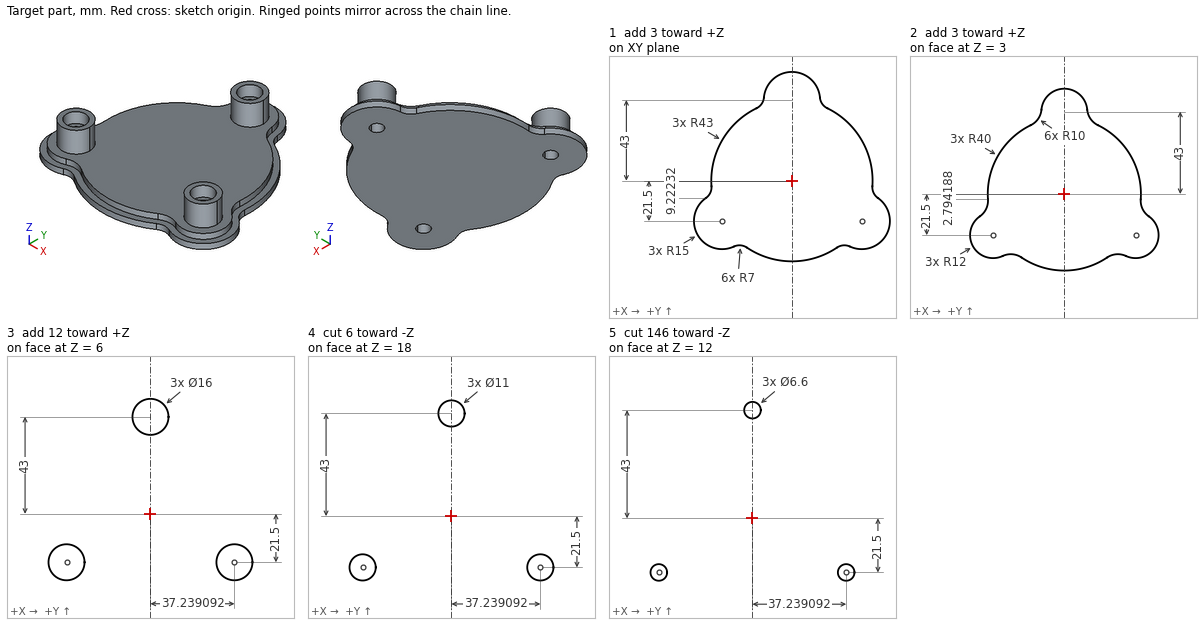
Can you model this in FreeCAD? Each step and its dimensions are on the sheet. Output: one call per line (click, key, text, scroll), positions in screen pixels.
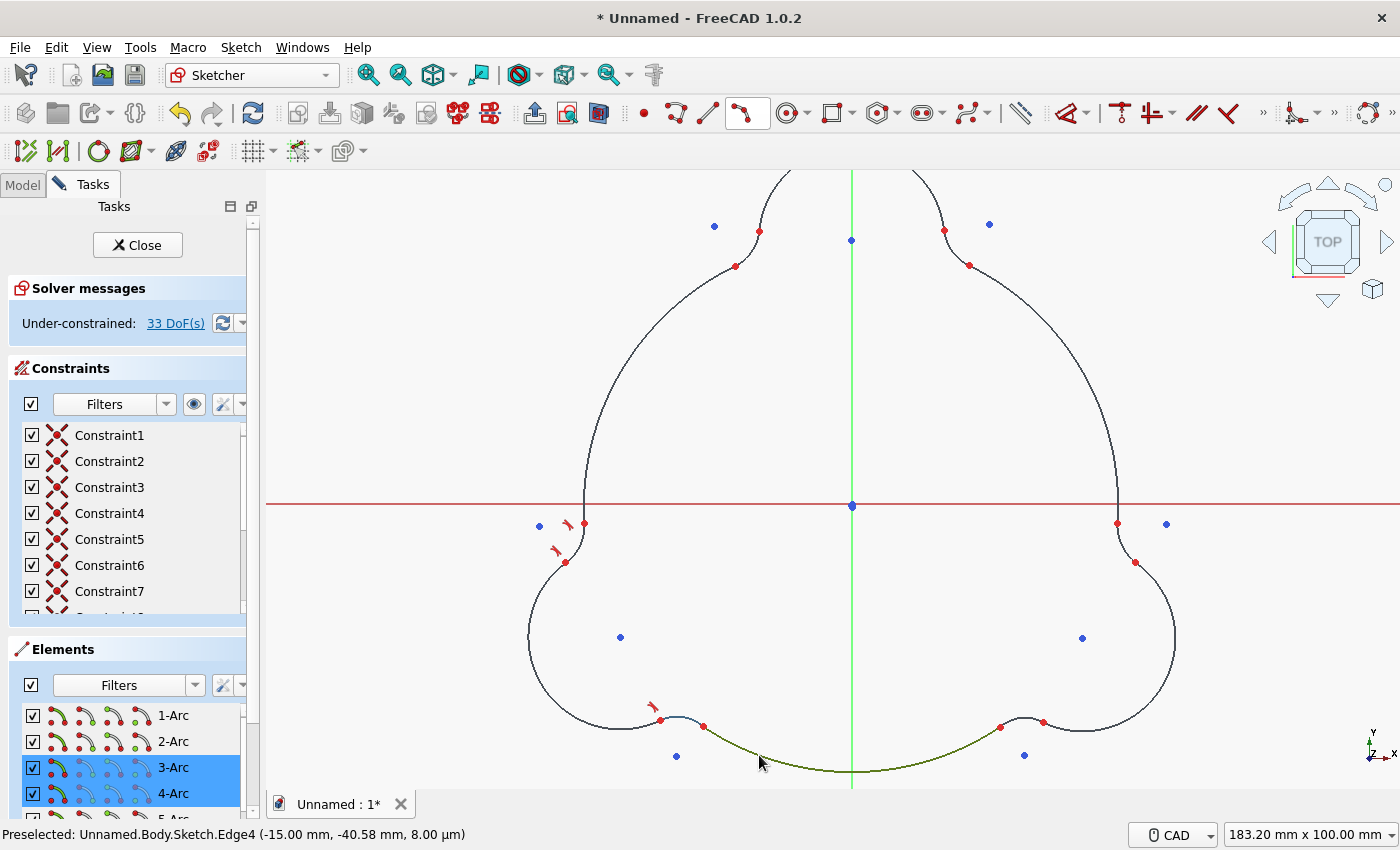
key(t)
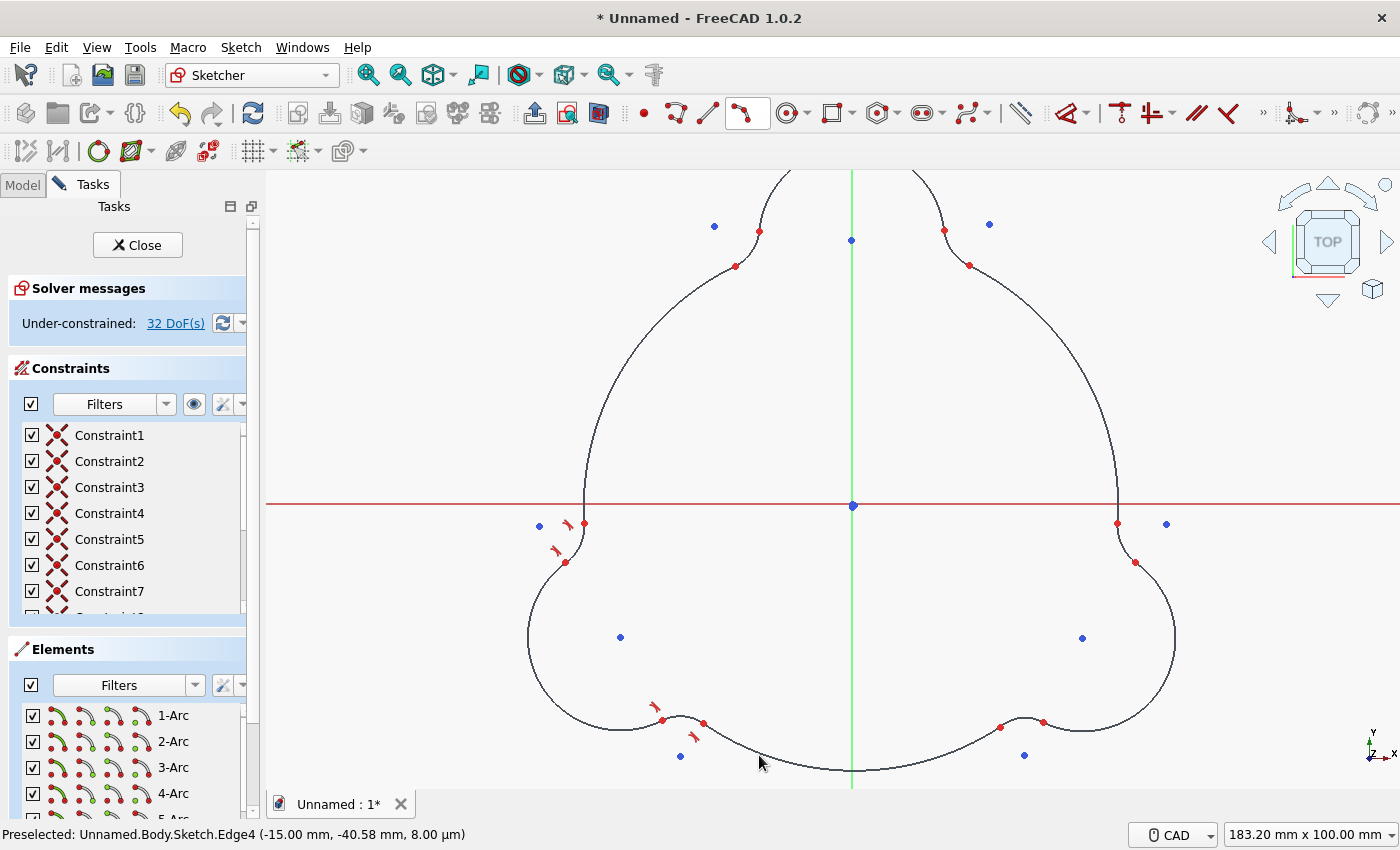
click(759, 753)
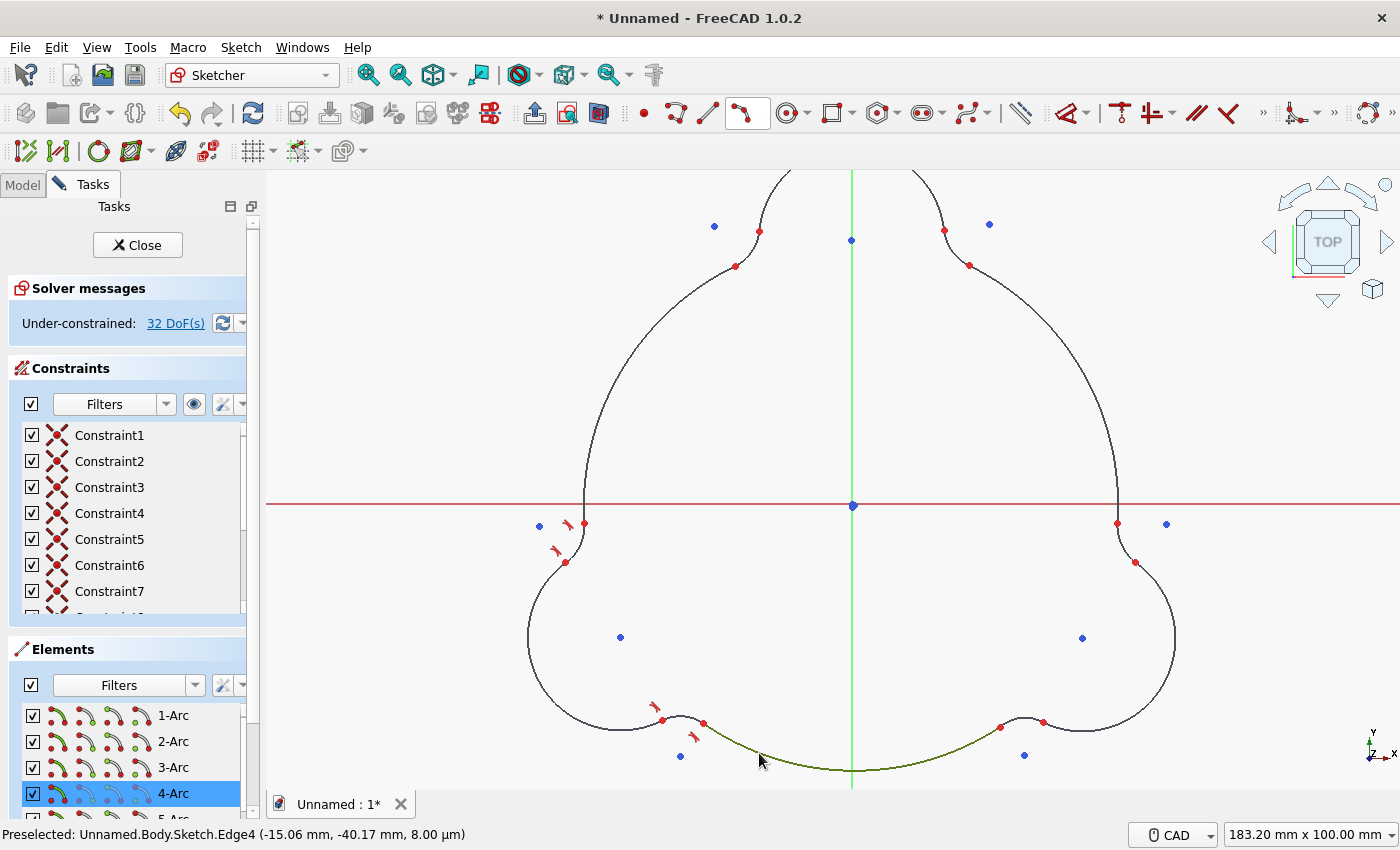
click(1030, 718)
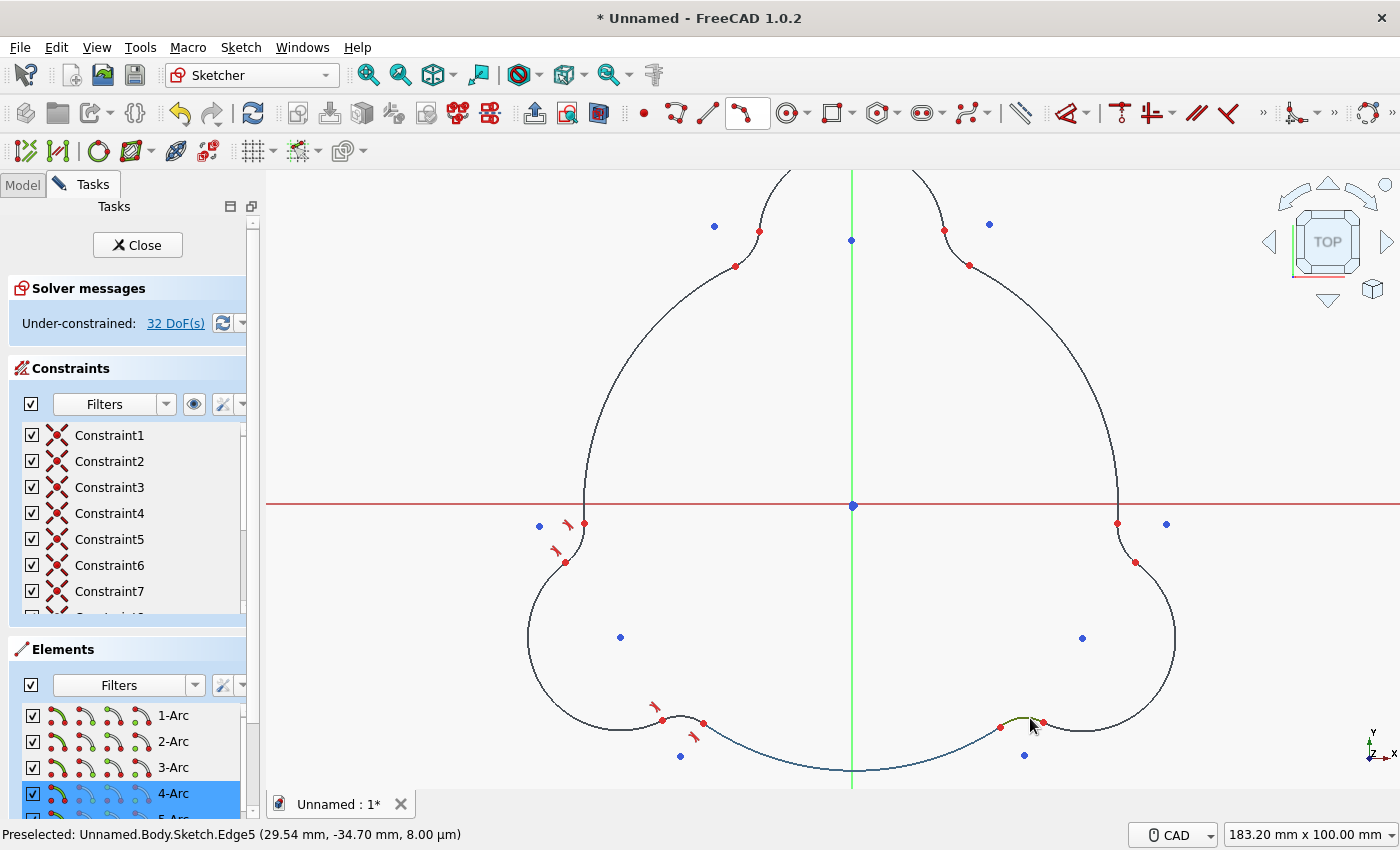
key(t)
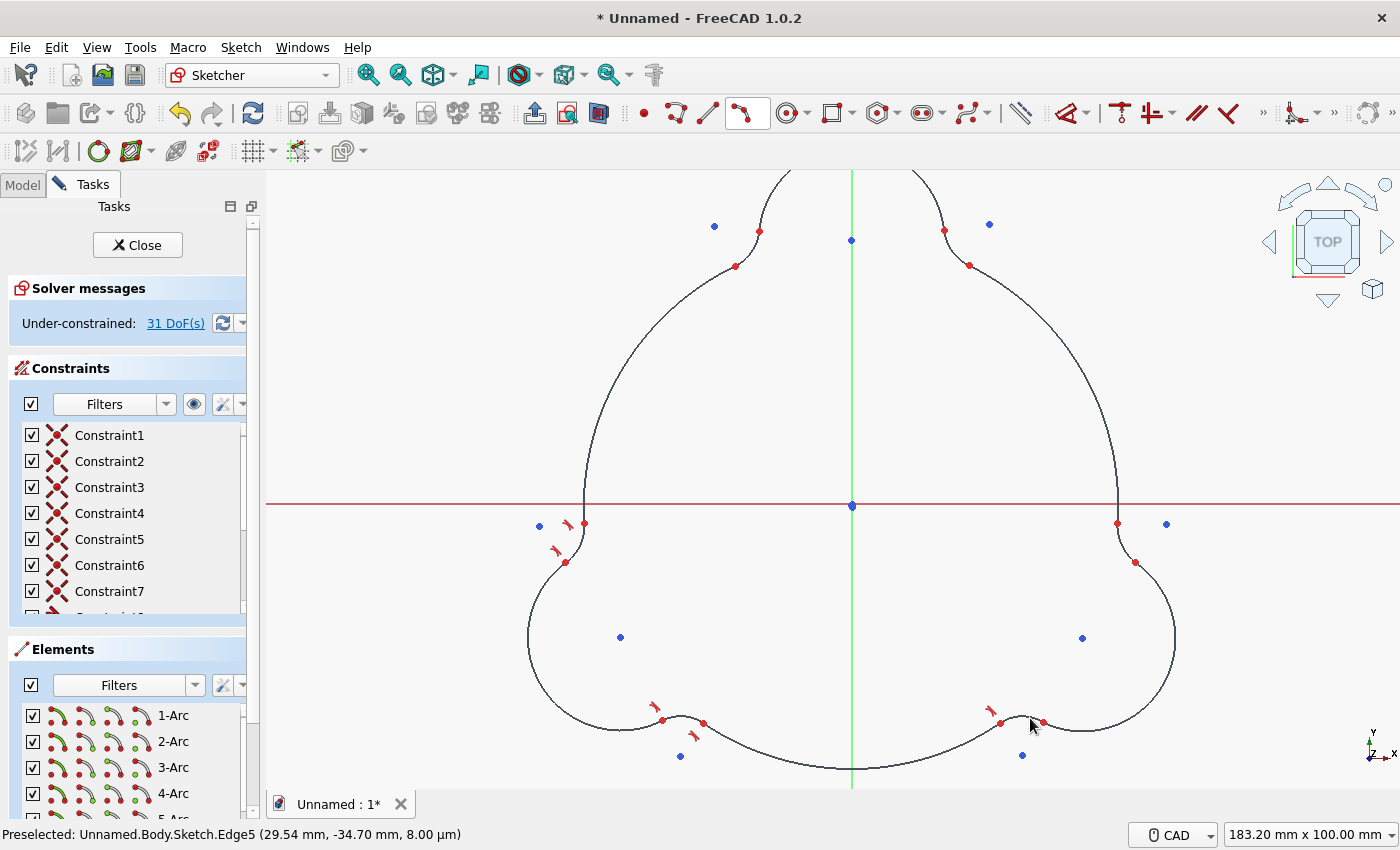
click(1031, 717)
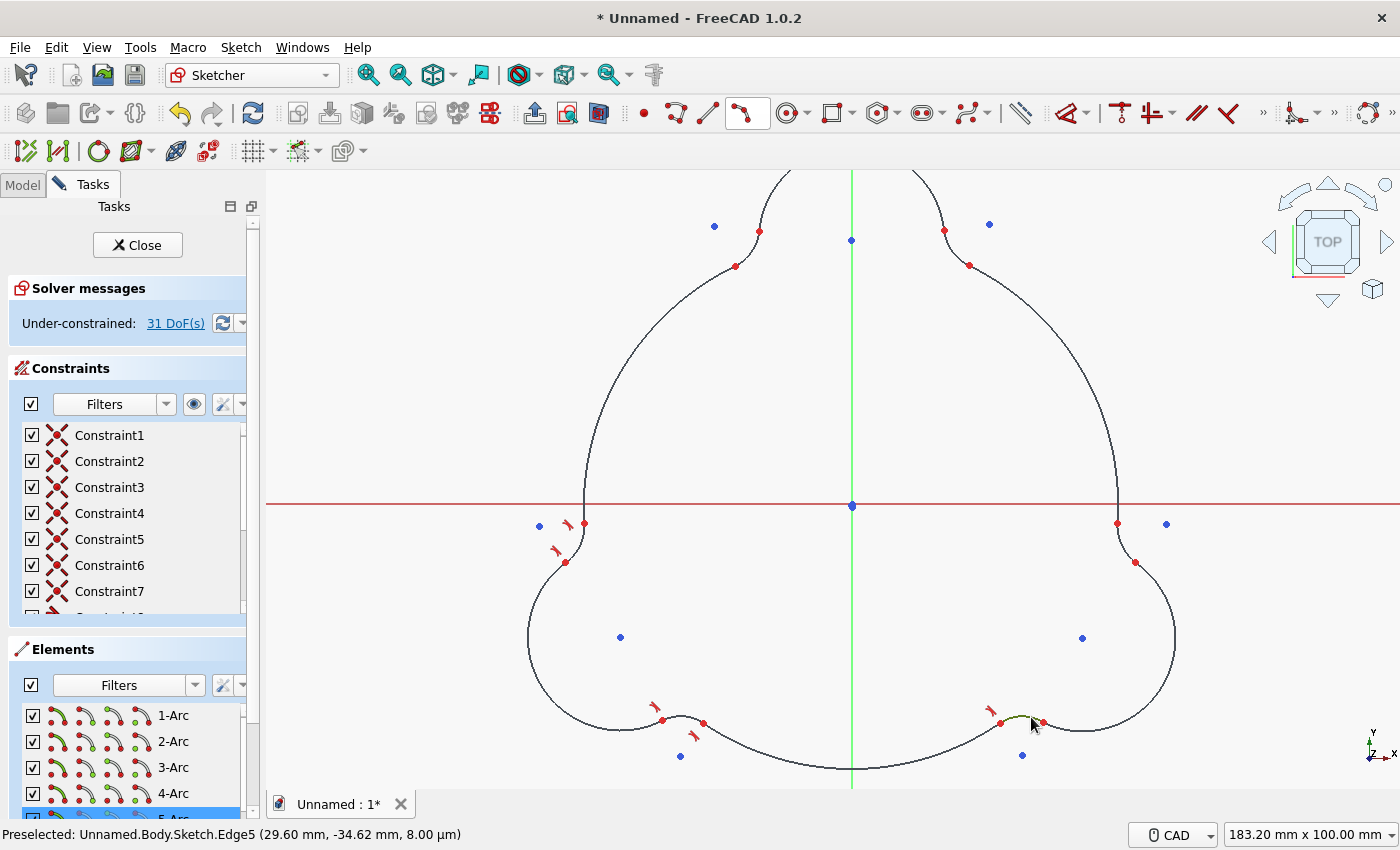
click(1123, 722)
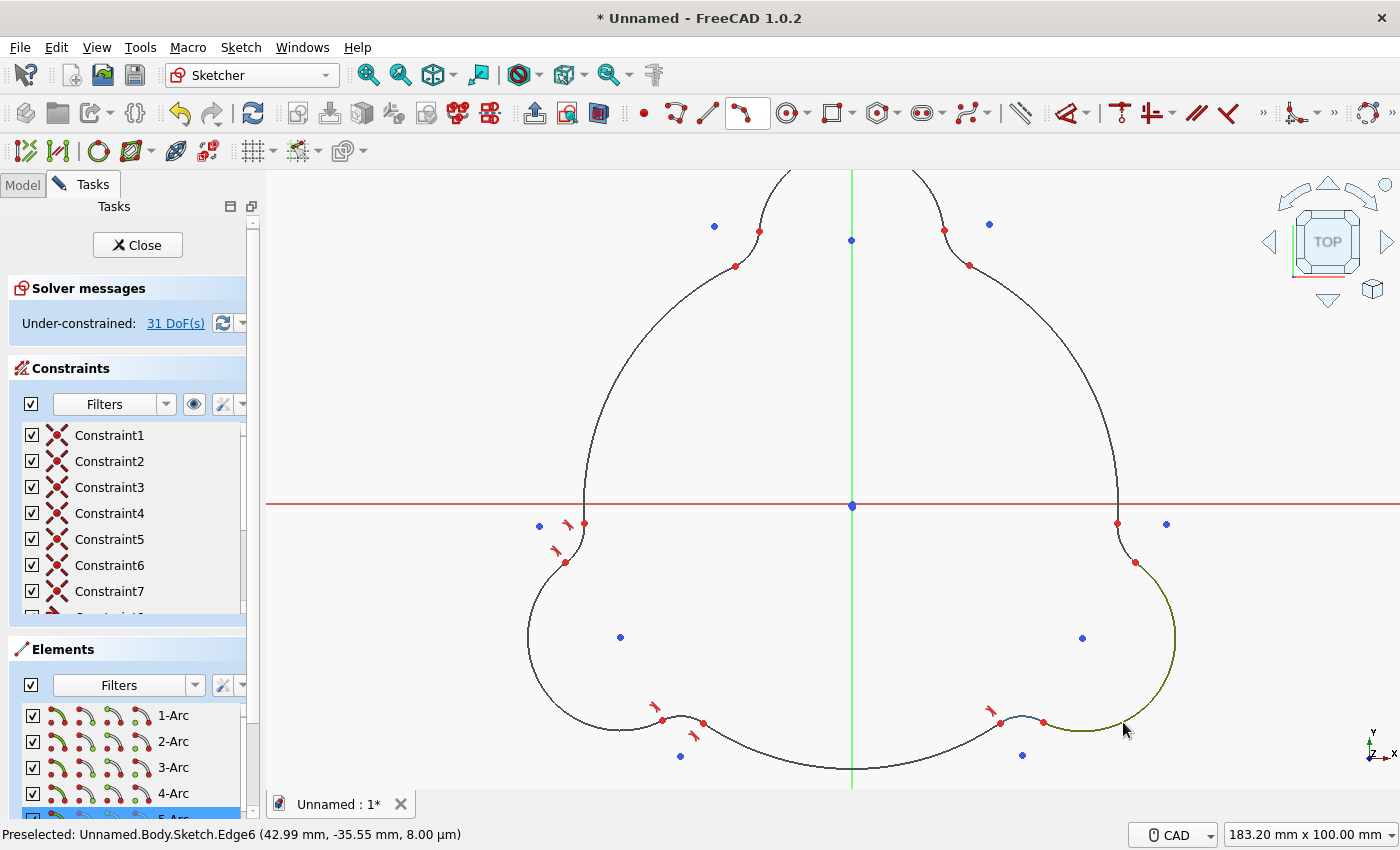
key(t)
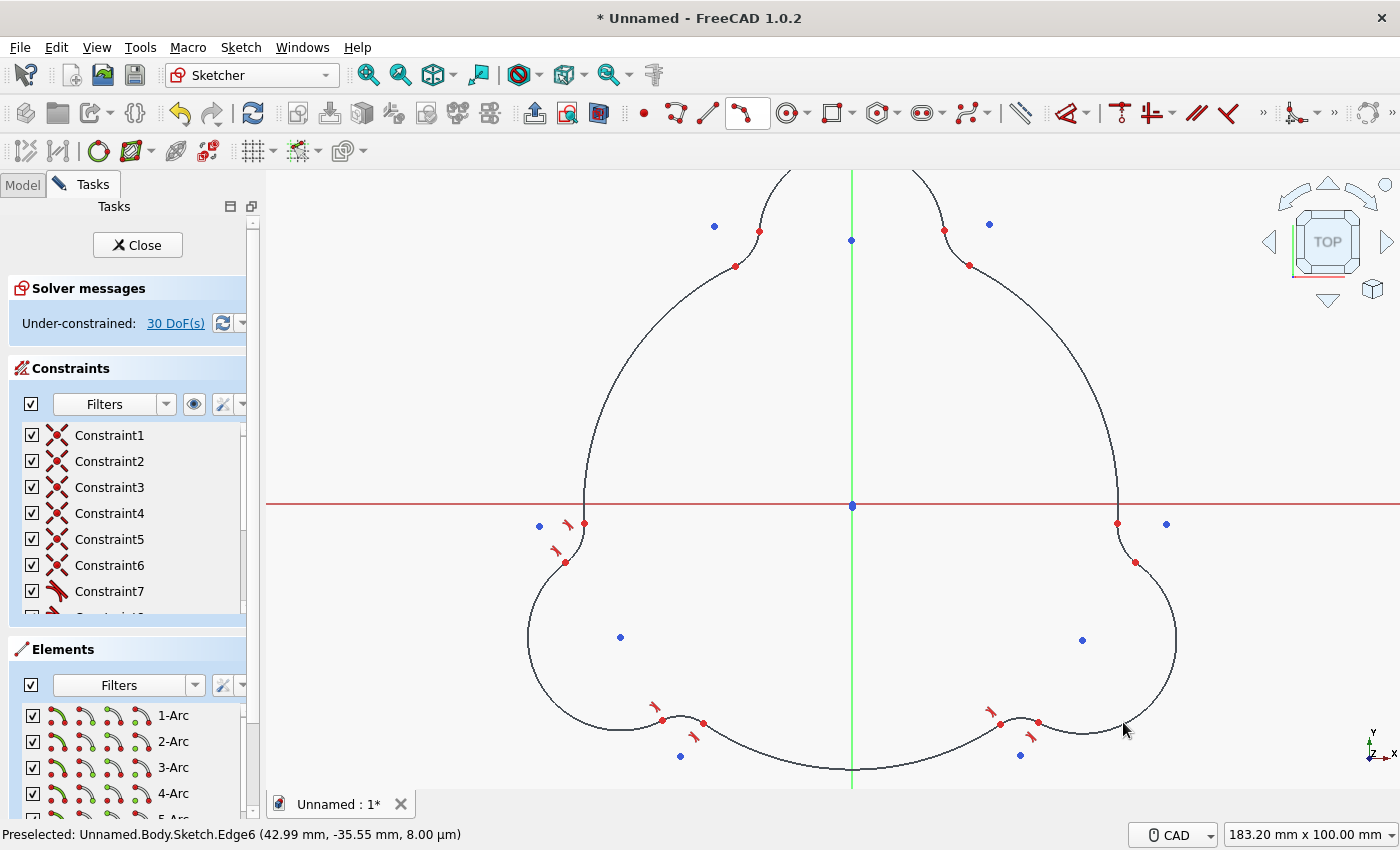
click(1121, 726)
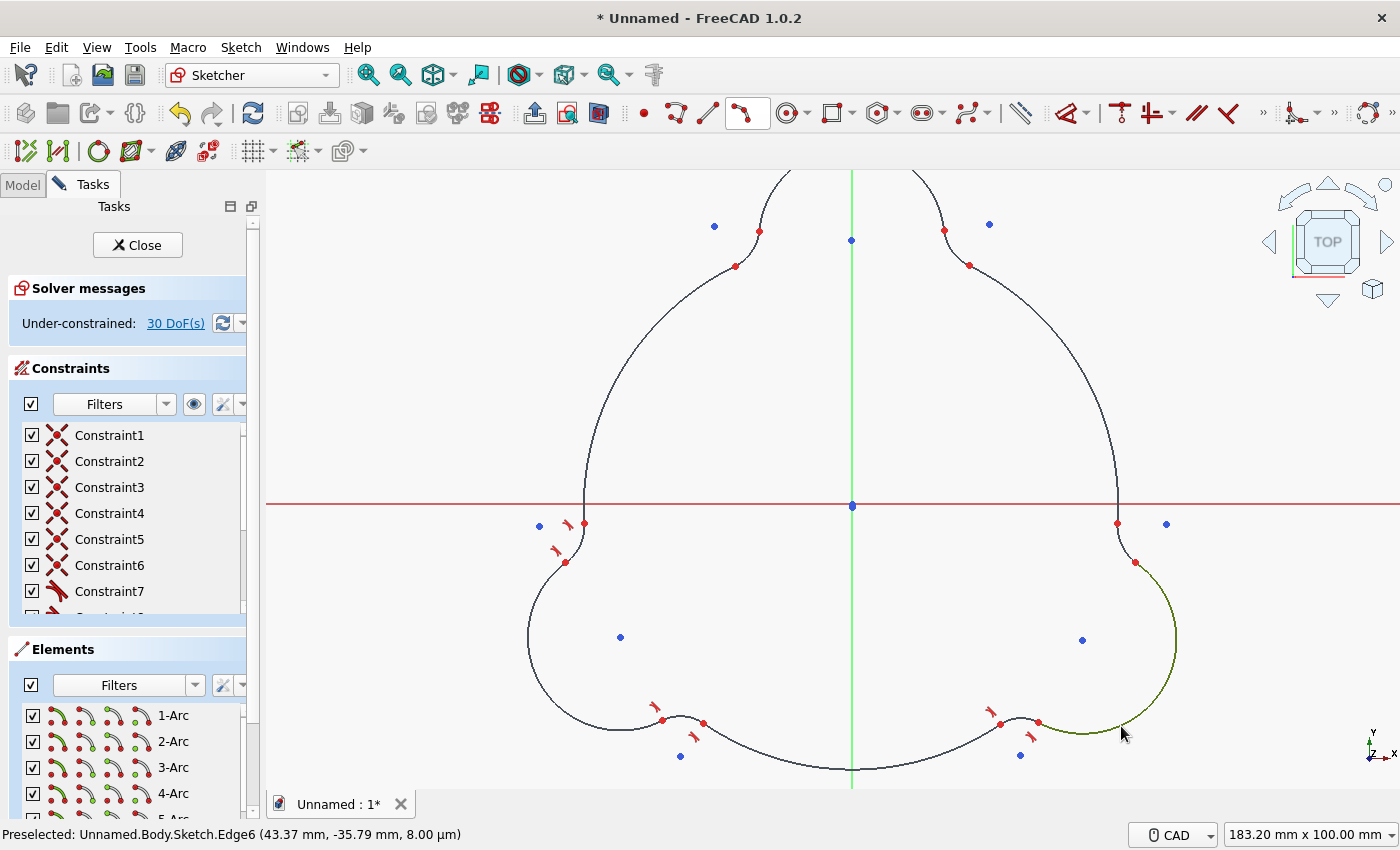
click(1119, 537)